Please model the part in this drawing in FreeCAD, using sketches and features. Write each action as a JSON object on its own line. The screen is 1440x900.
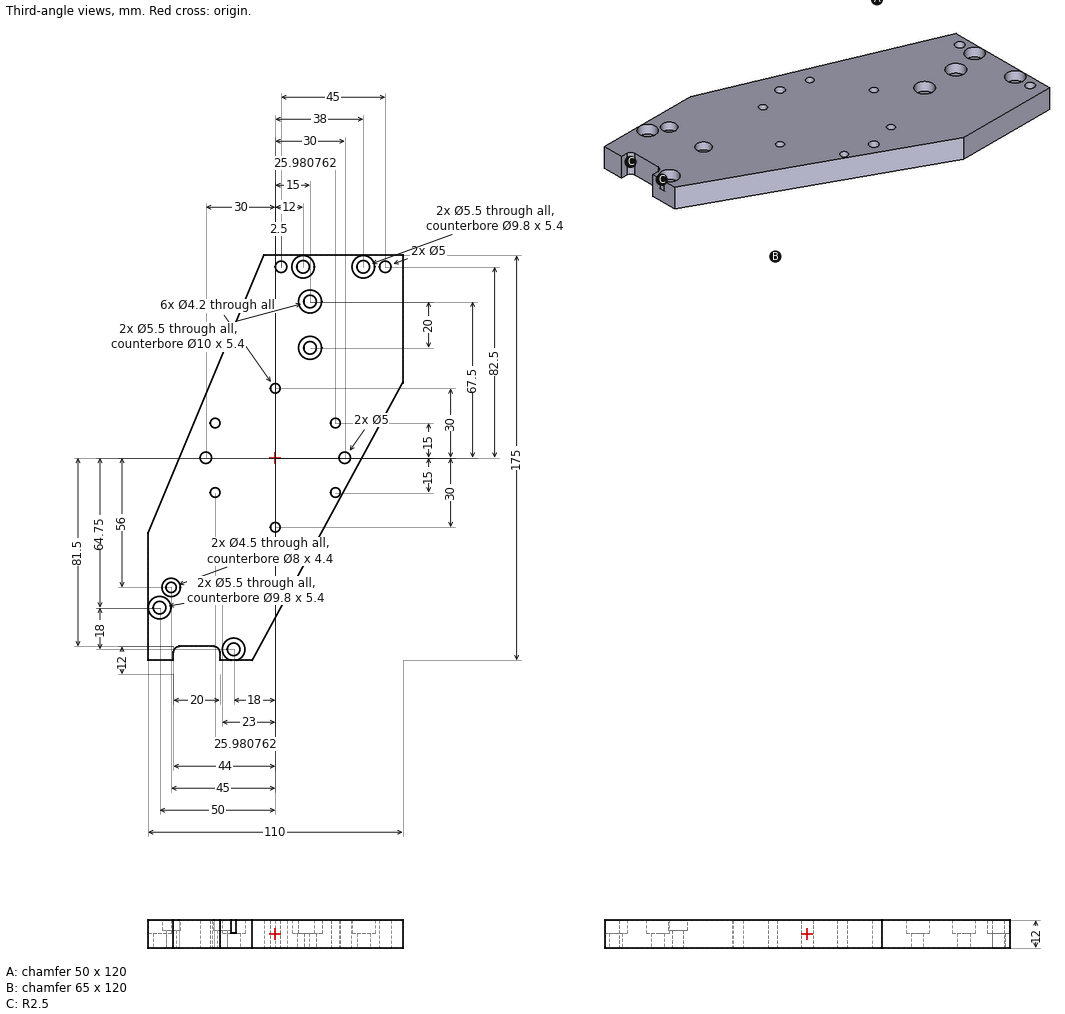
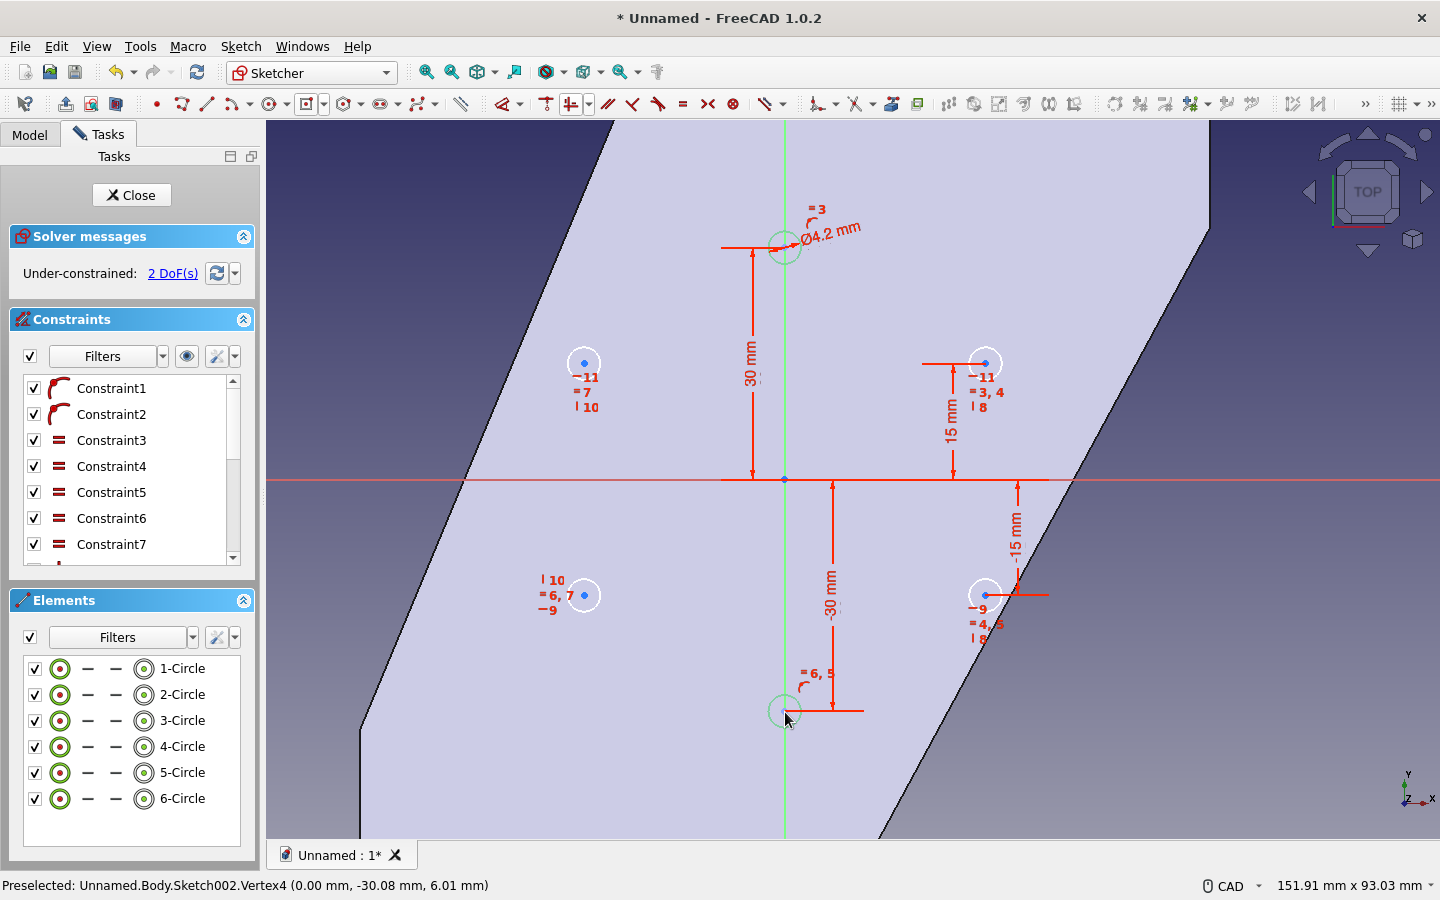
{"action": "left_click", "coordinate": [986, 364]}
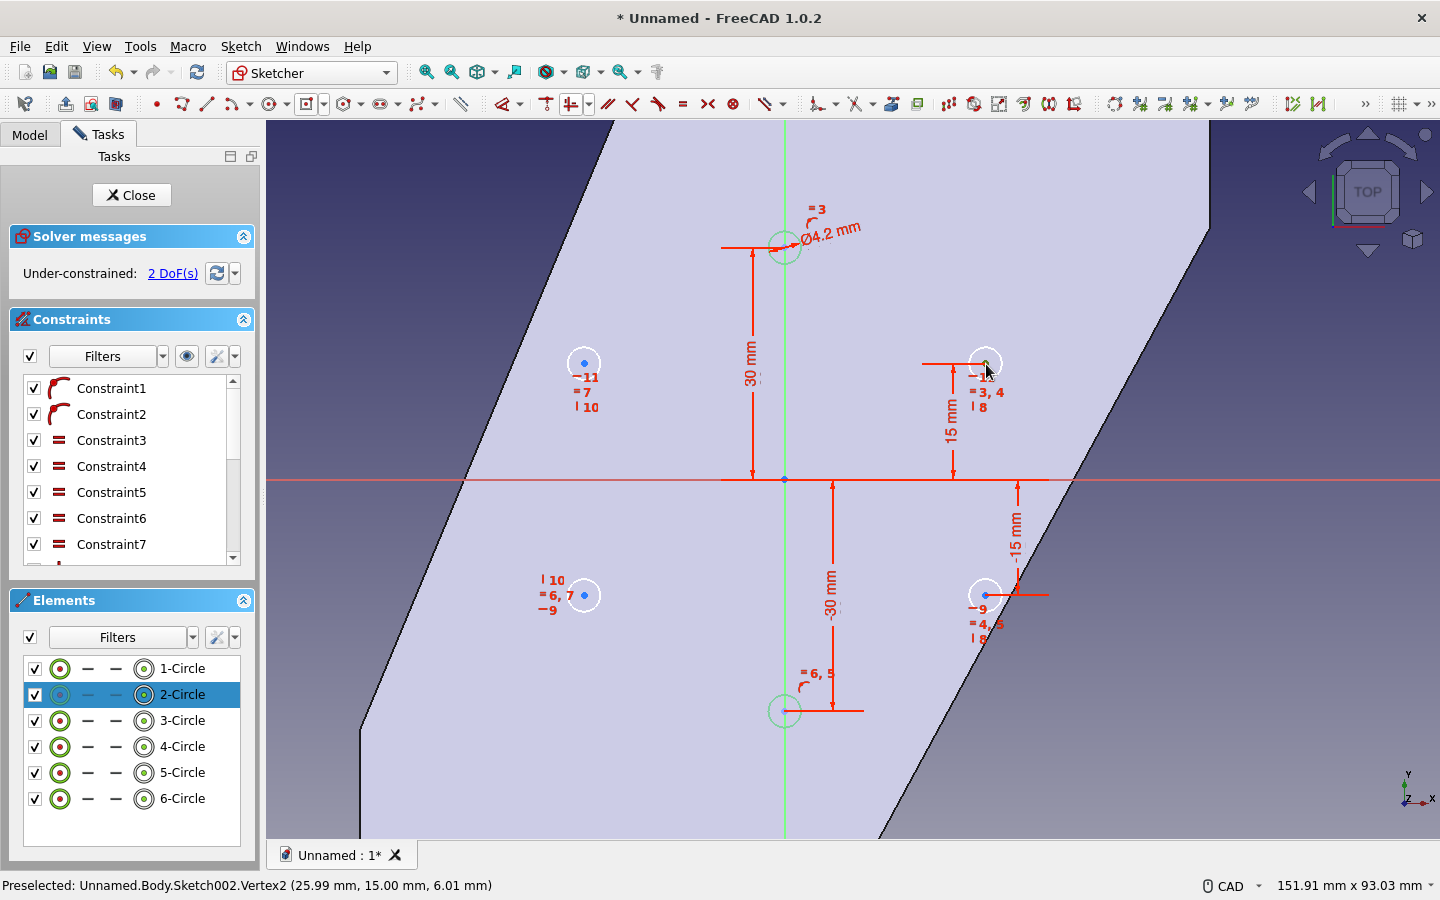
{"action": "key", "text": "l"}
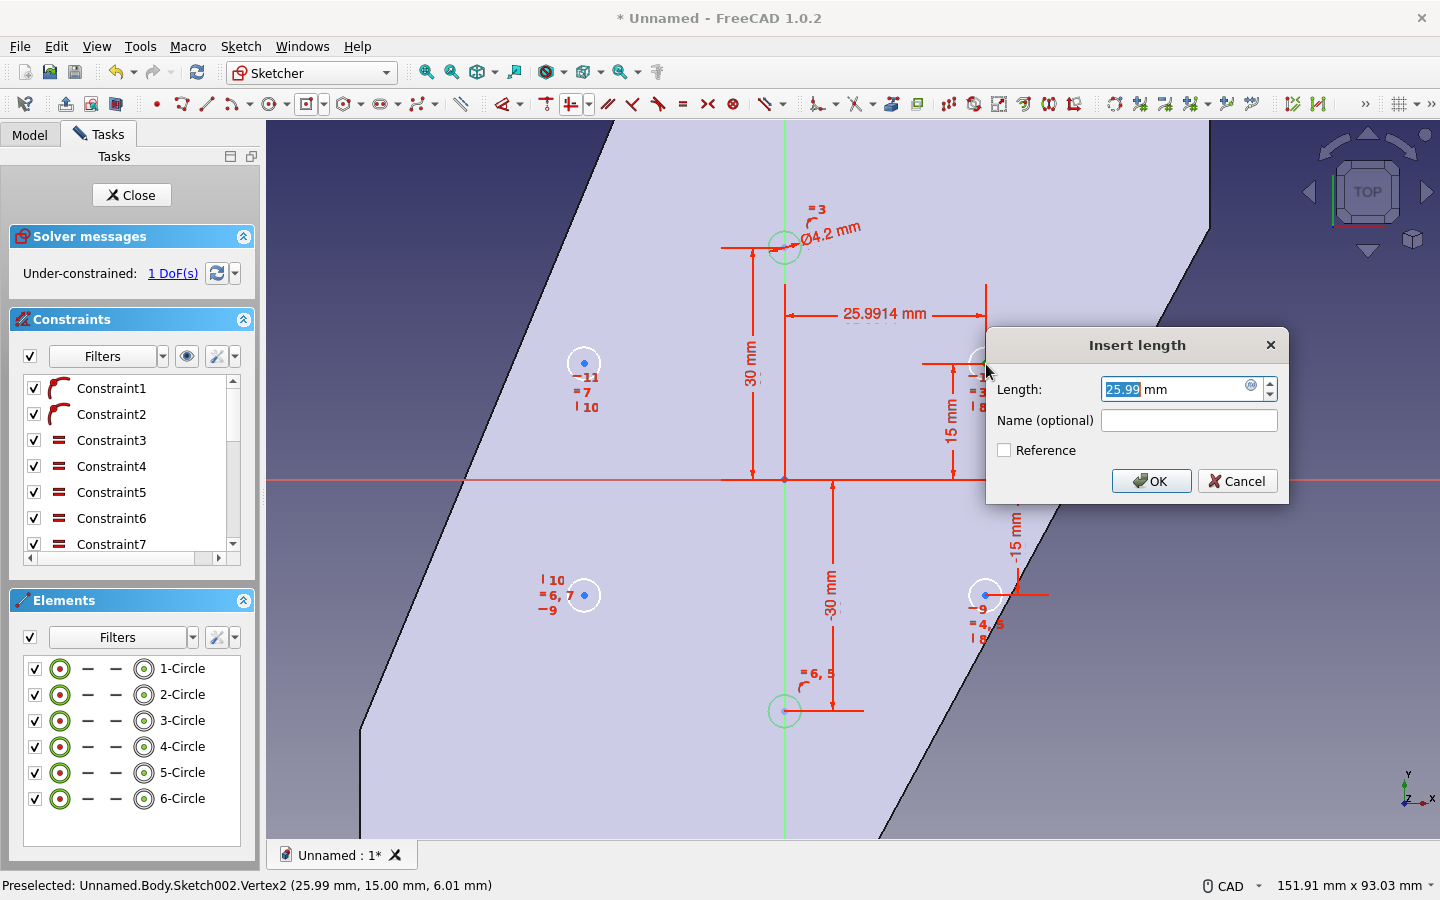
{"action": "type", "text": "25.980762"}
{"action": "key", "text": "Return"}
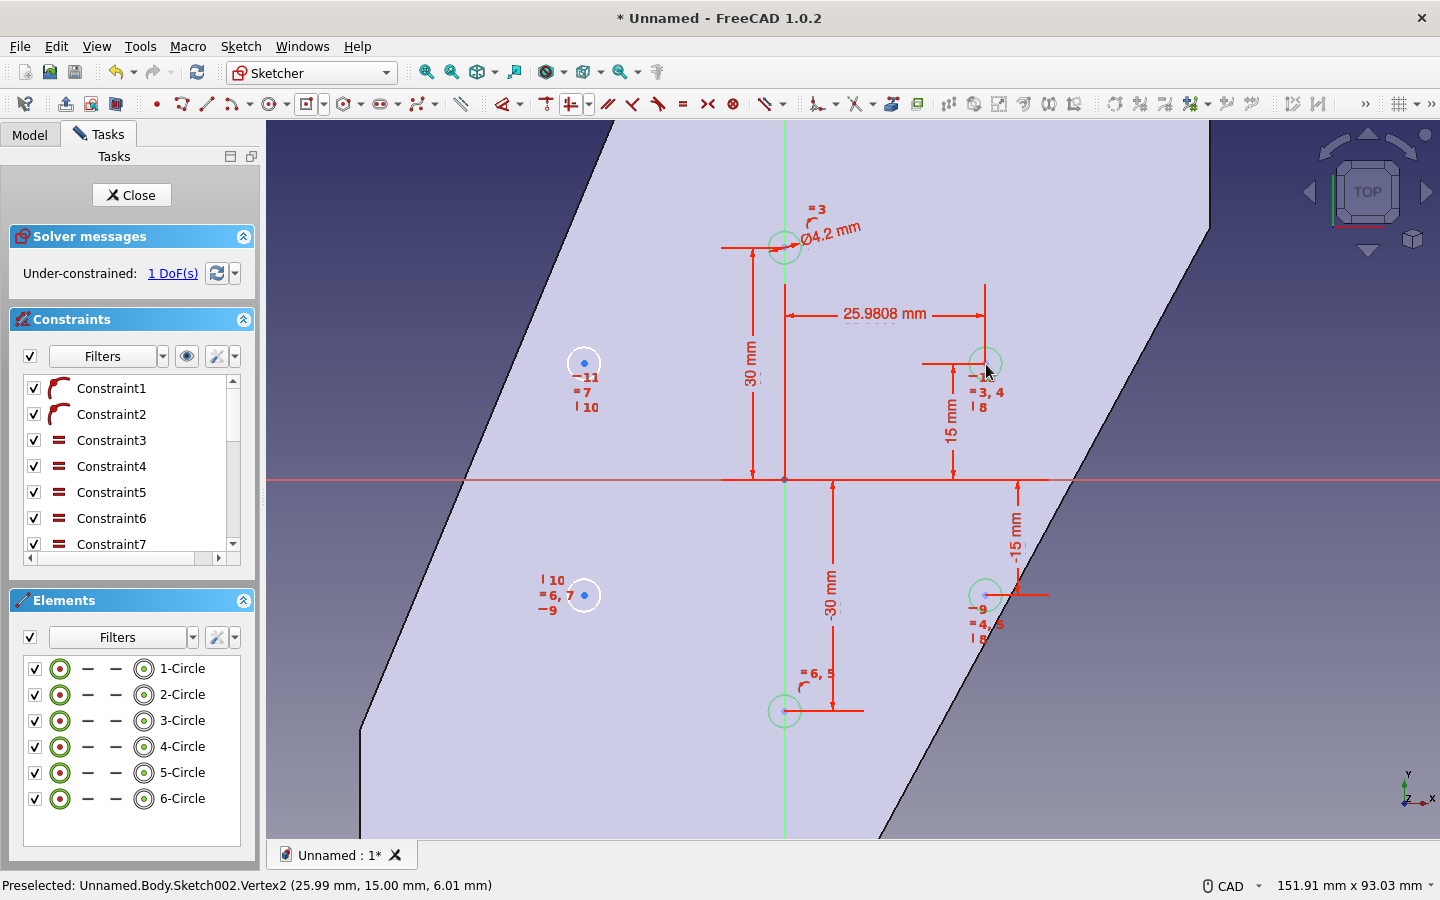
{"action": "left_click", "coordinate": [584, 595]}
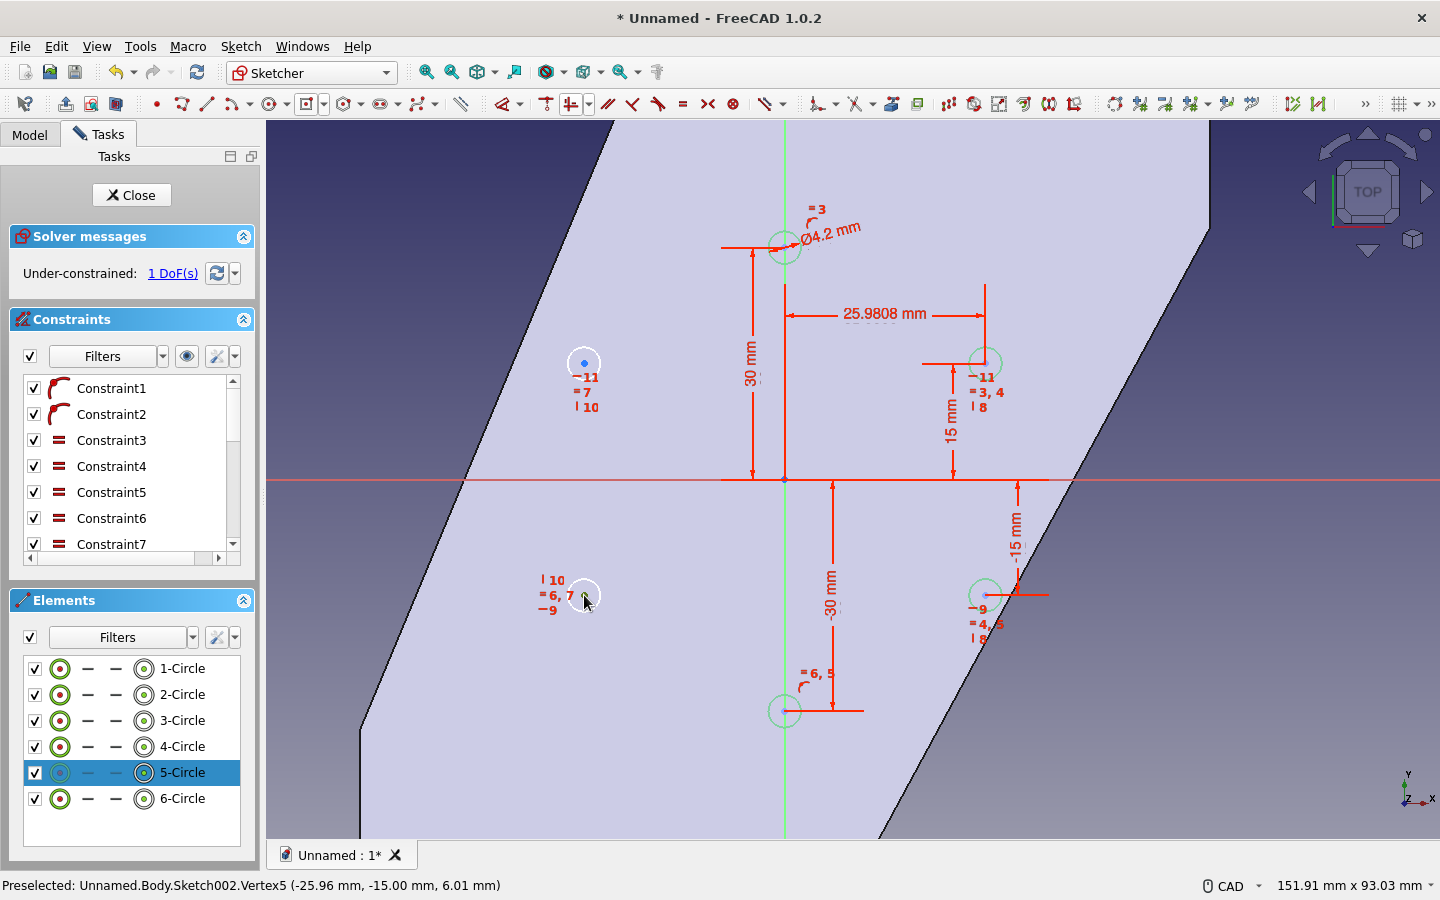
{"action": "key", "text": "l"}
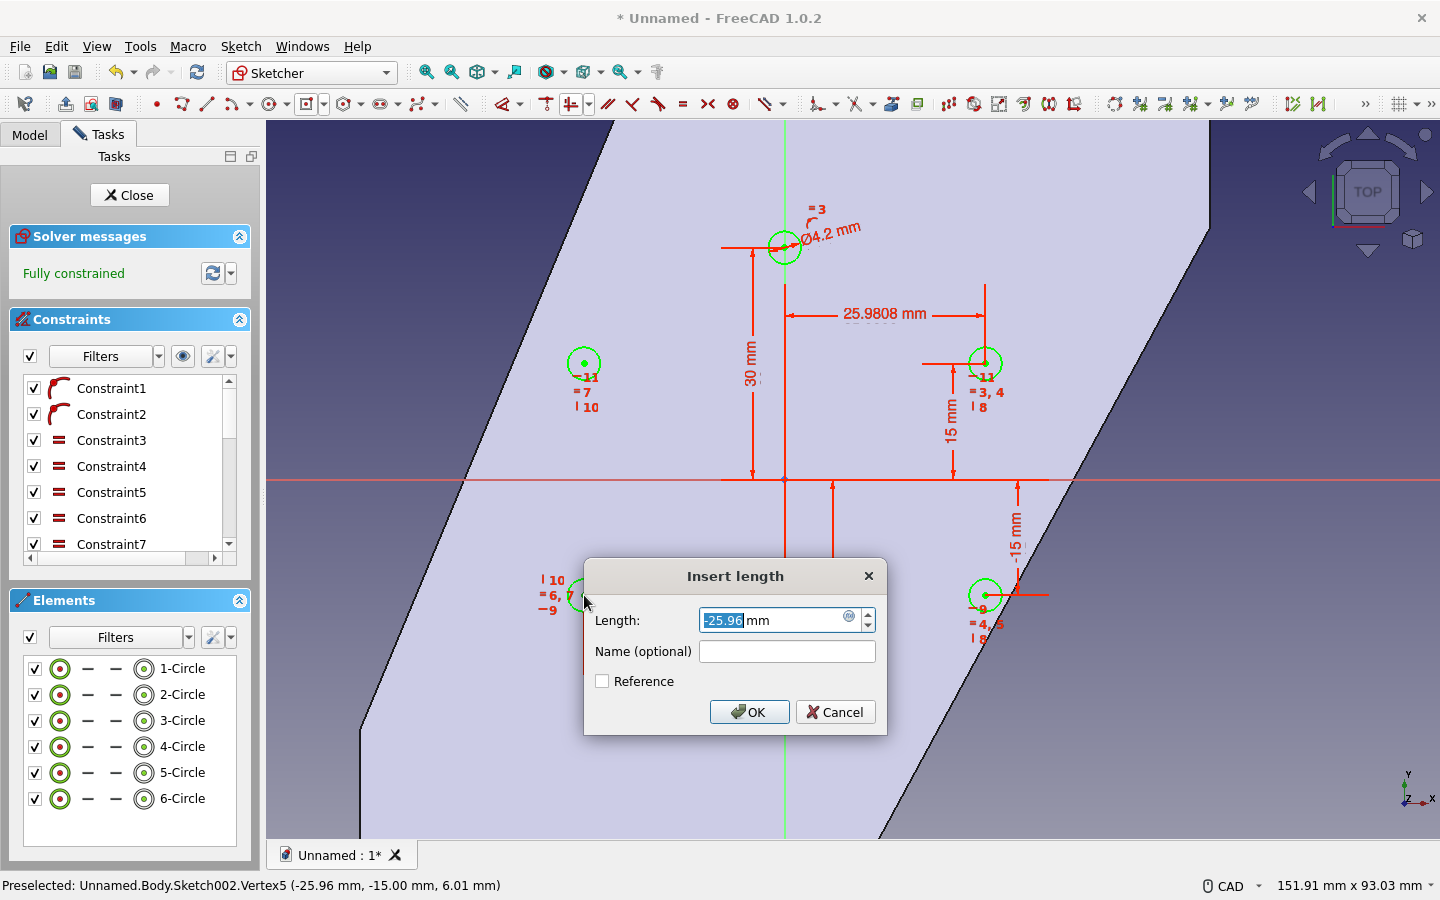
{"action": "type", "text": "-25.980762"}
{"action": "key", "text": "Return"}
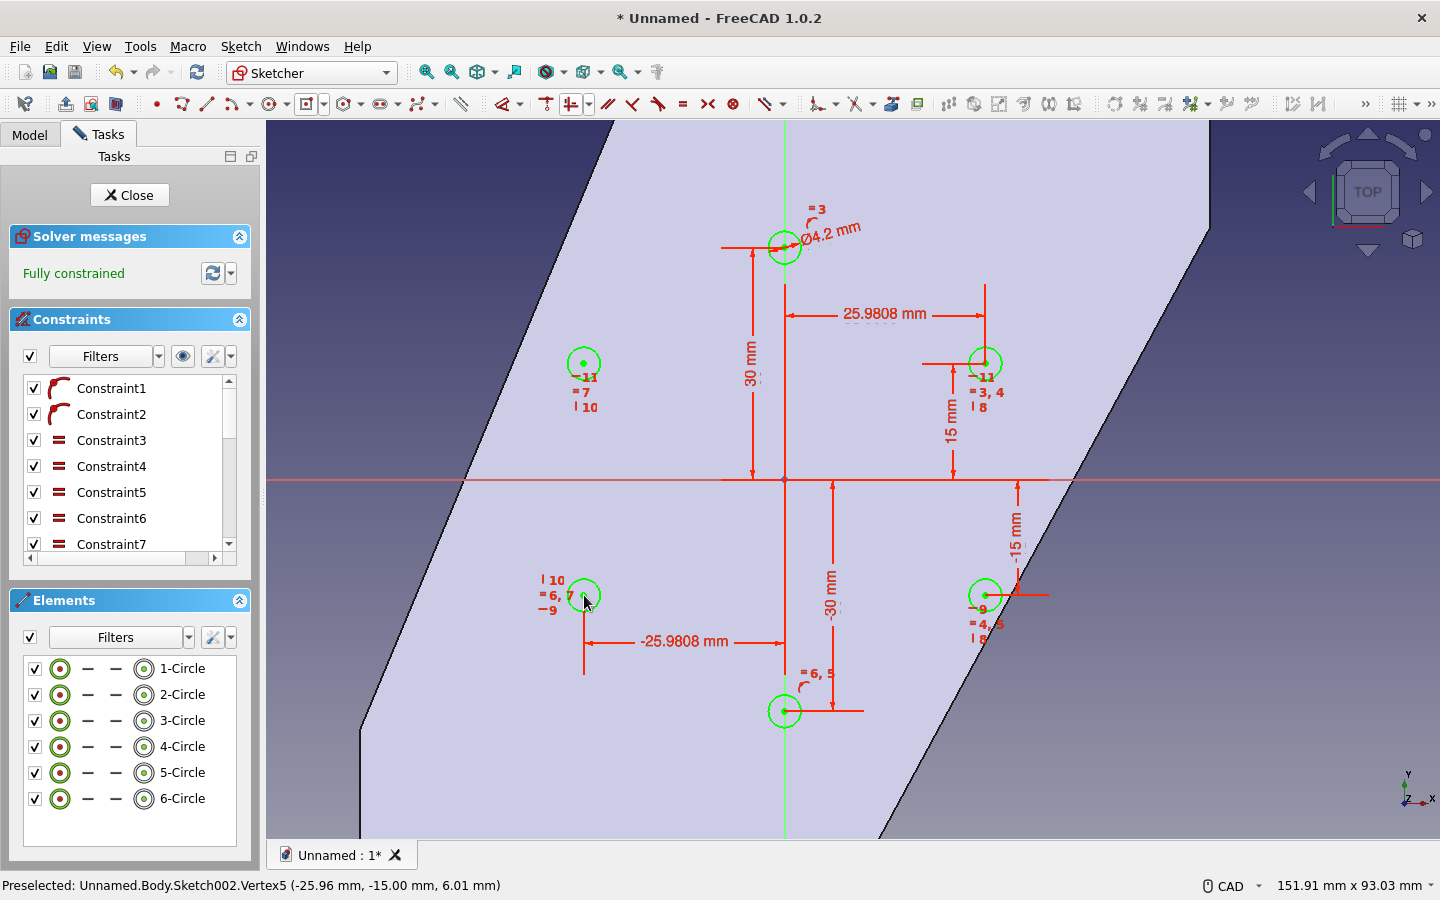
{"action": "left_click", "coordinate": [130, 195]}